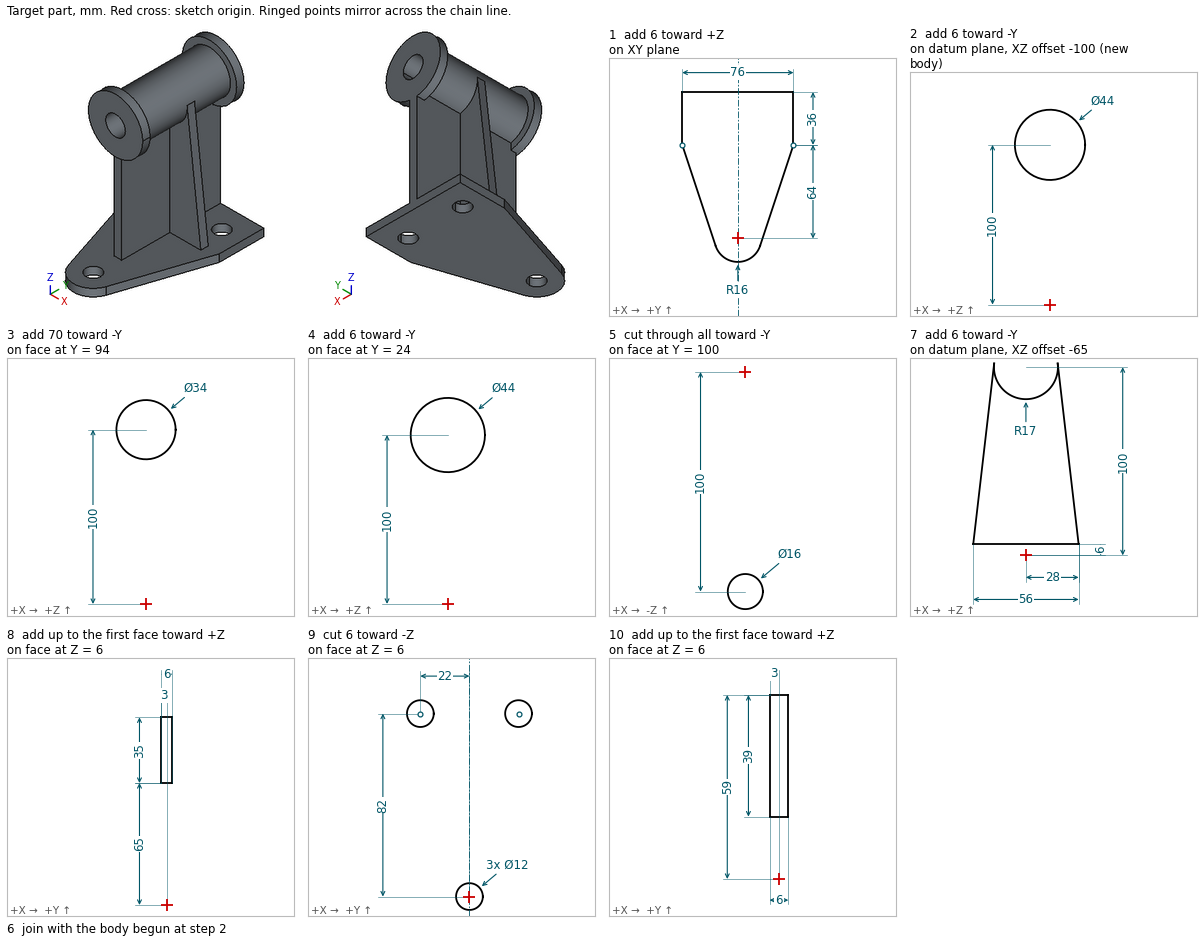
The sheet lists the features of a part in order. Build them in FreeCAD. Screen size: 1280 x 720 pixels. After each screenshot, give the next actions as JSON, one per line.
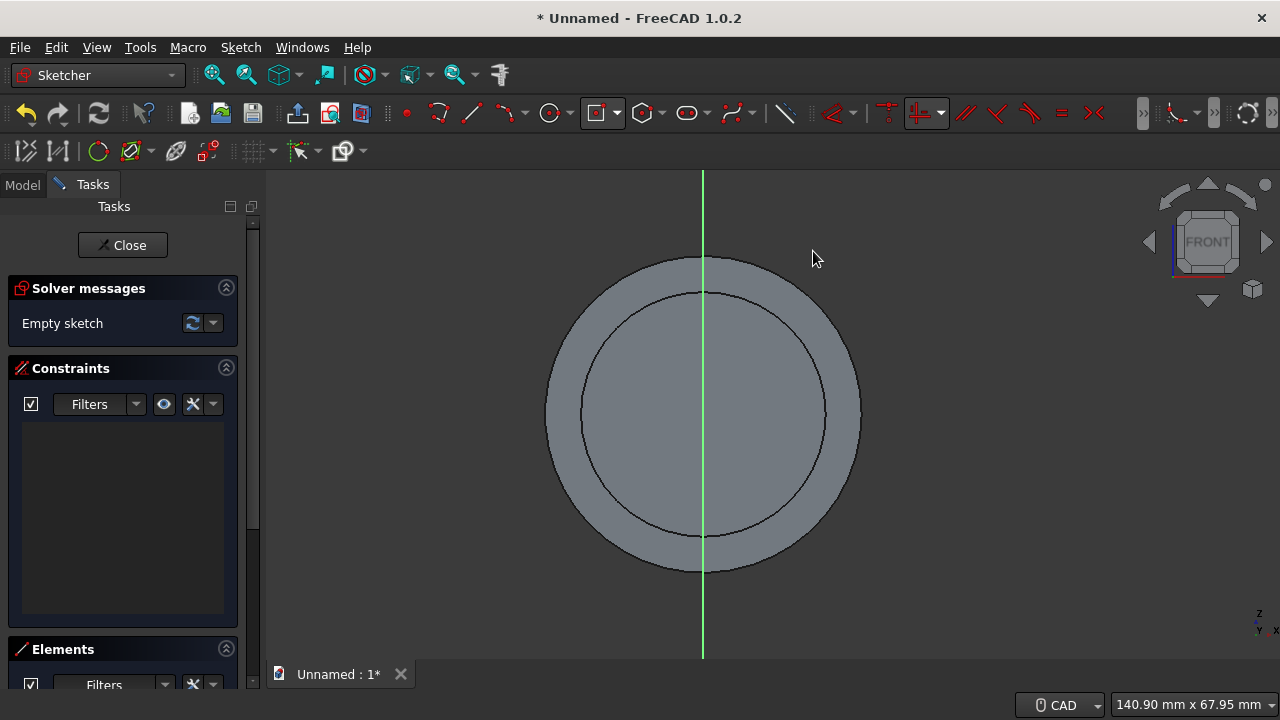
{"action": "key", "text": "g c"}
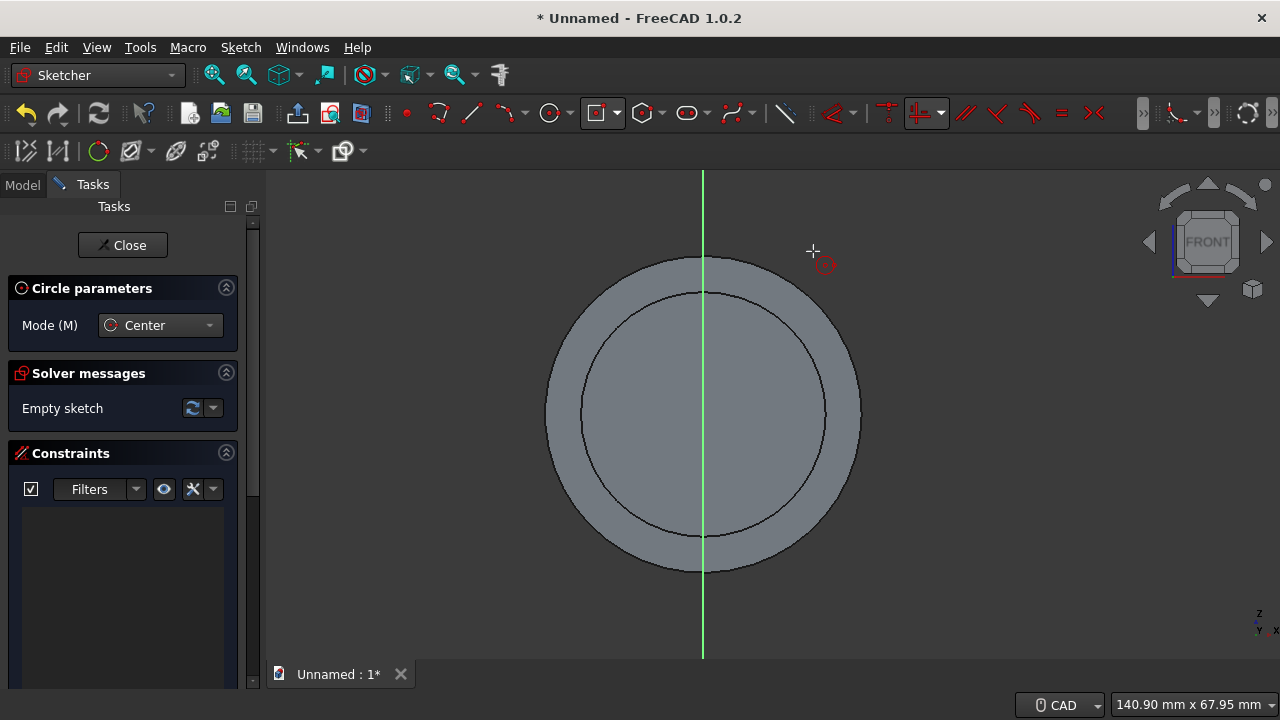
{"action": "left_click", "coordinate": [703, 414]}
{"action": "left_click", "coordinate": [815, 302]}
{"action": "key", "text": "Escape"}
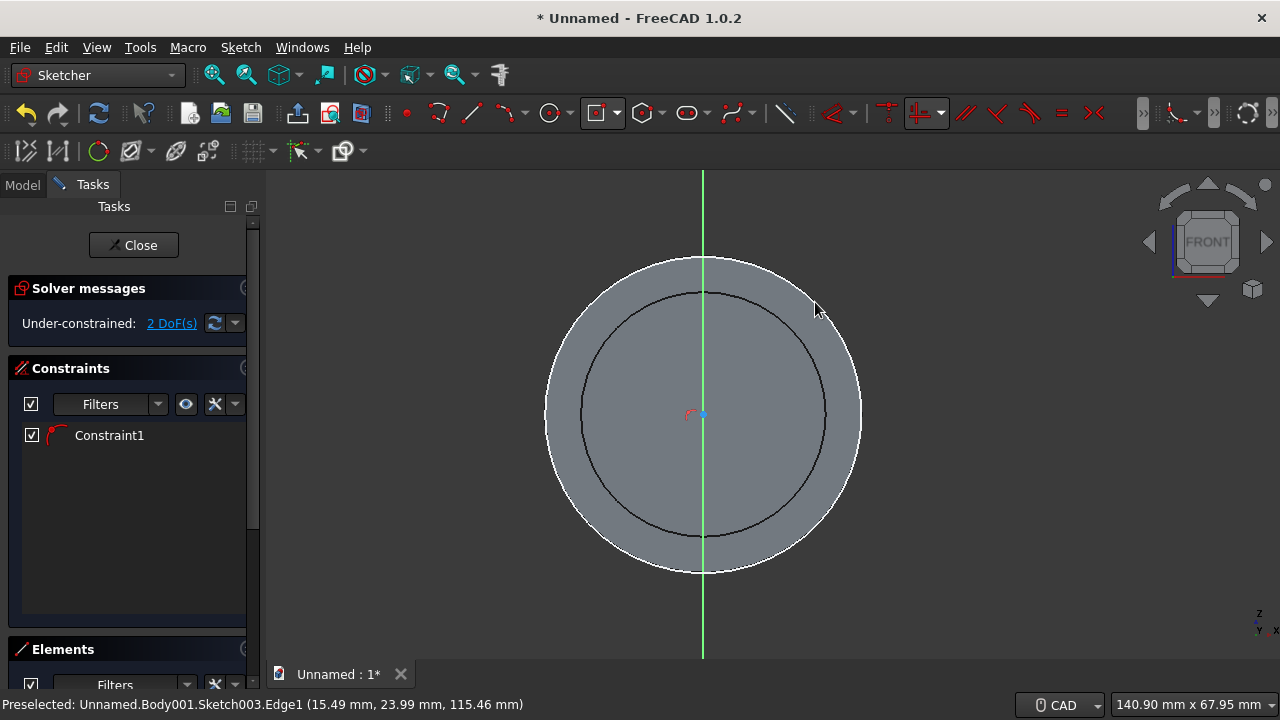
{"action": "key", "text": "d"}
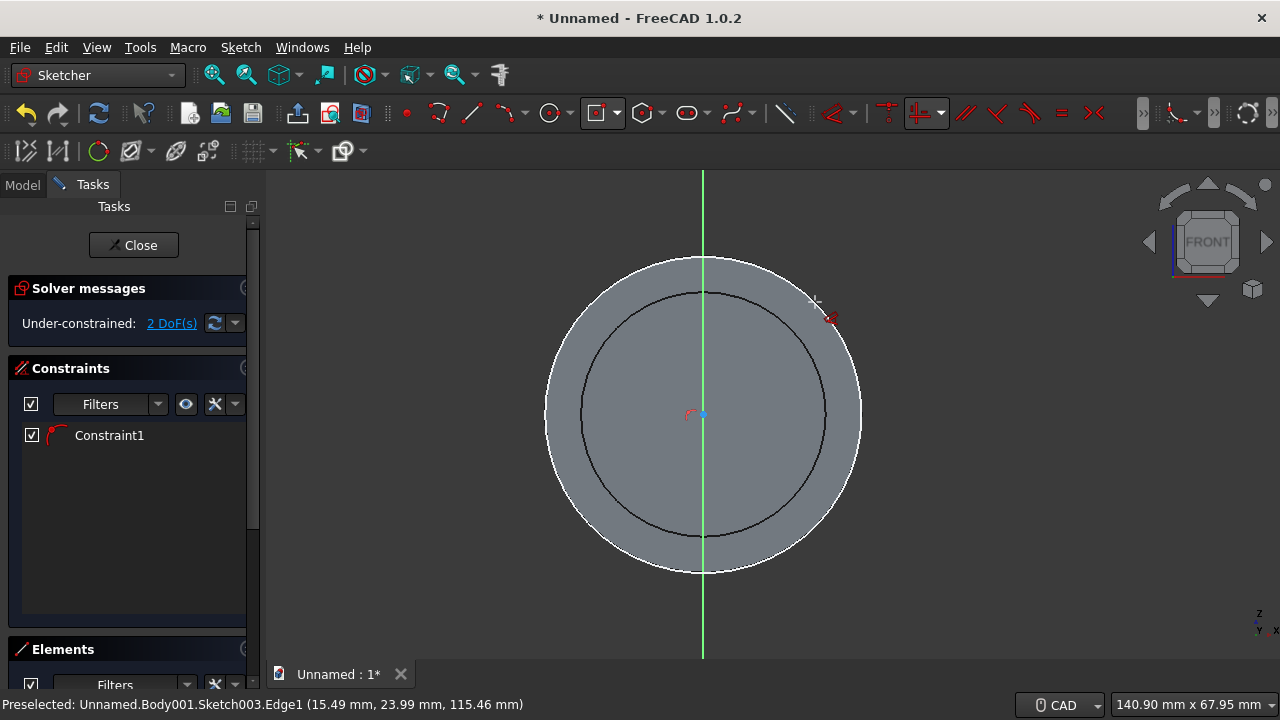
{"action": "left_click", "coordinate": [815, 303]}
{"action": "left_click", "coordinate": [838, 280]}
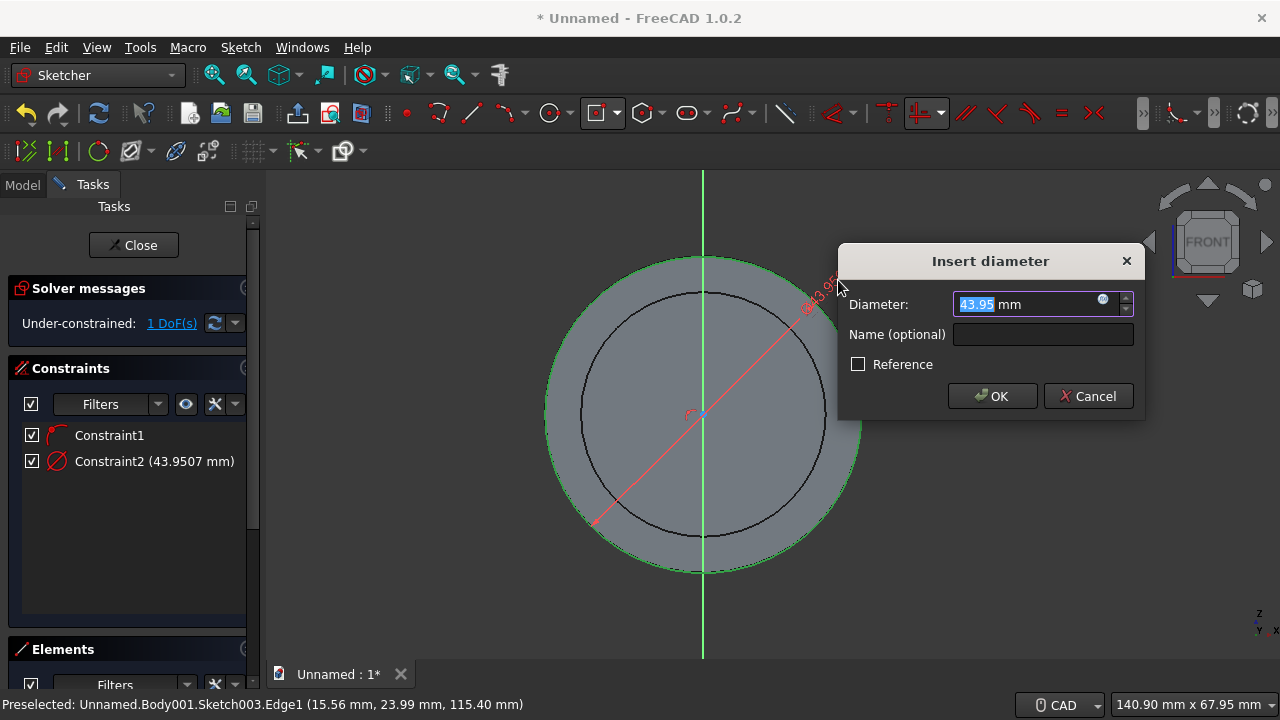
{"action": "type", "text": "44"}
{"action": "key", "text": "Return"}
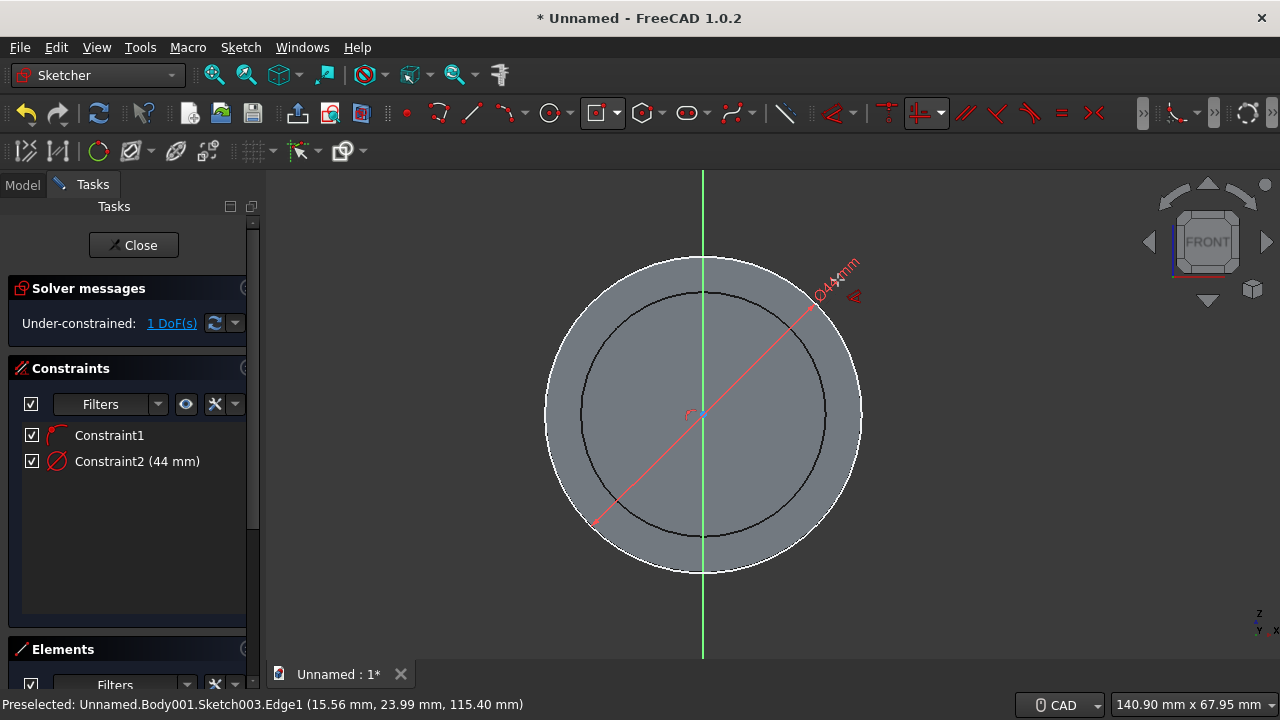
{"action": "left_click", "coordinate": [703, 415]}
{"action": "left_click", "coordinate": [737, 523]}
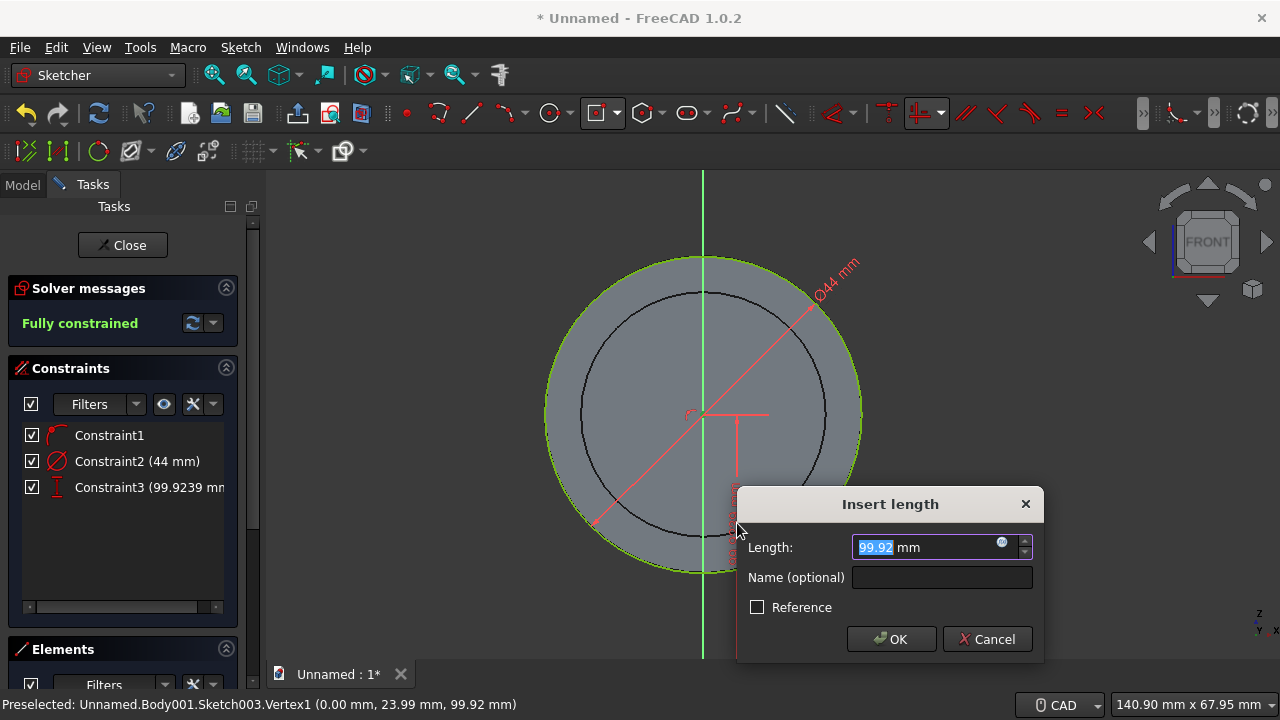
{"action": "type", "text": "100"}
{"action": "key", "text": "Return"}
{"action": "key", "text": "Escape"}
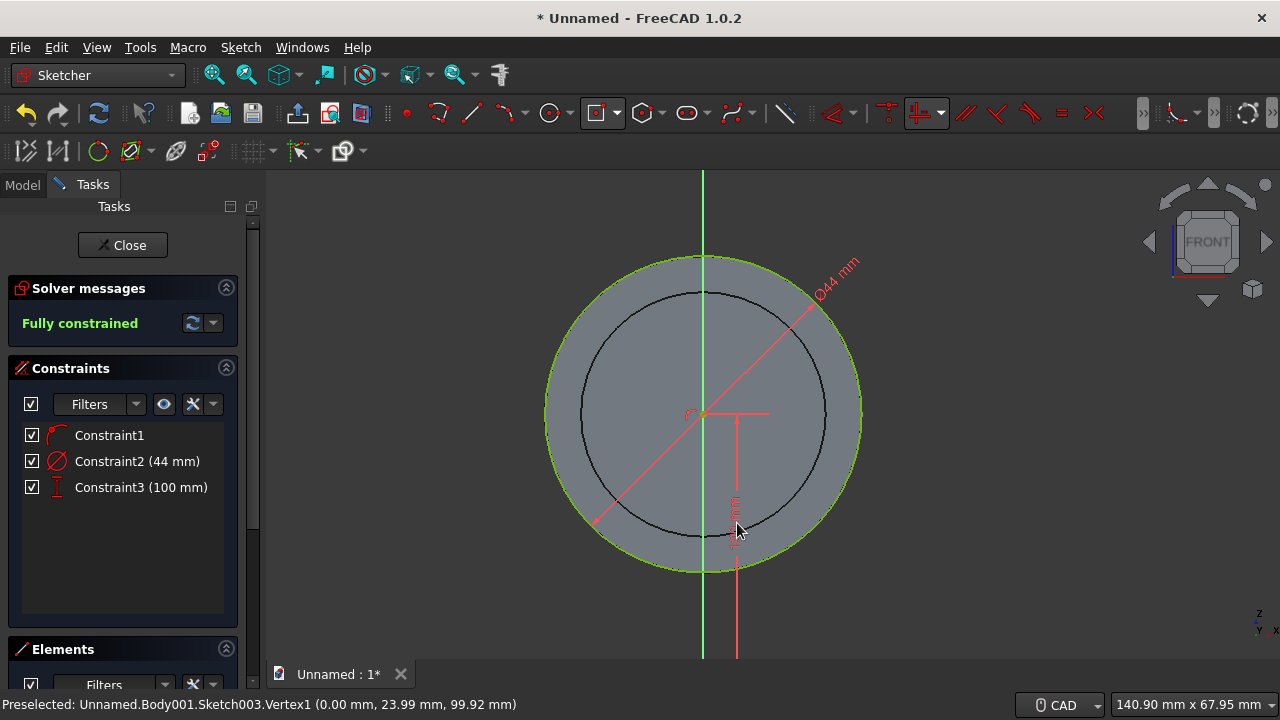
{"action": "left_click", "coordinate": [123, 245]}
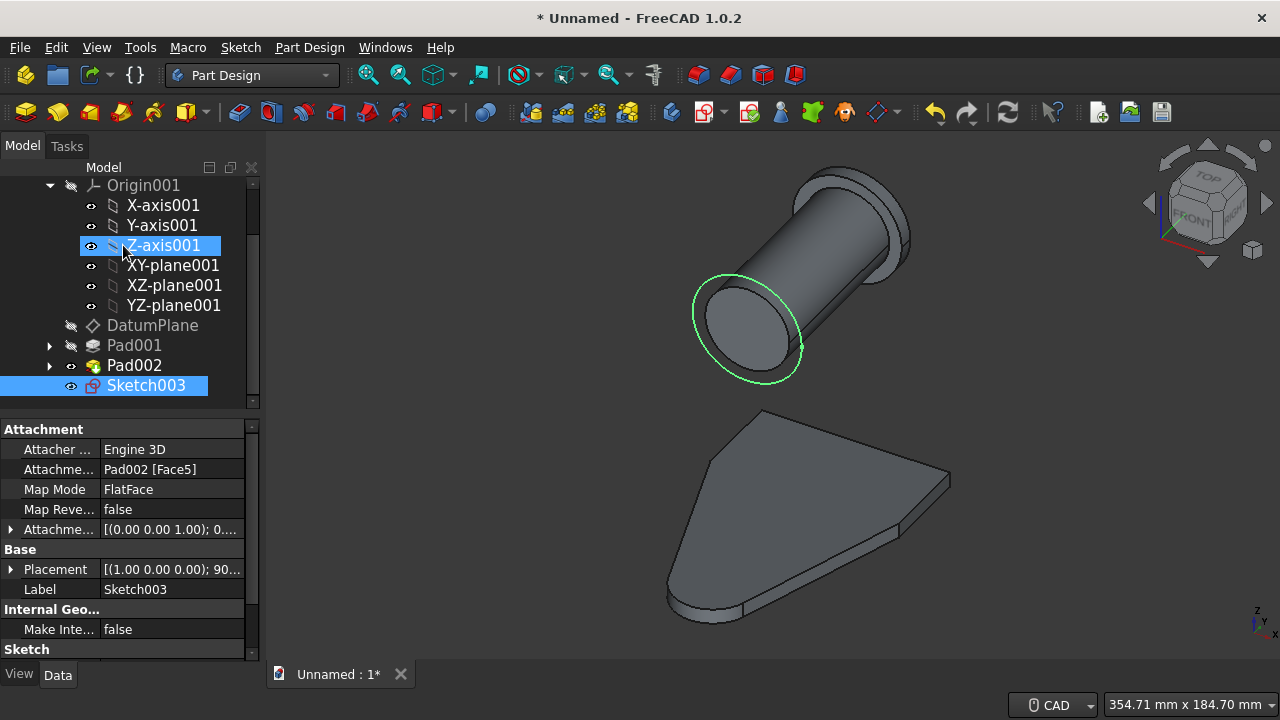
{"action": "left_click", "coordinate": [26, 112]}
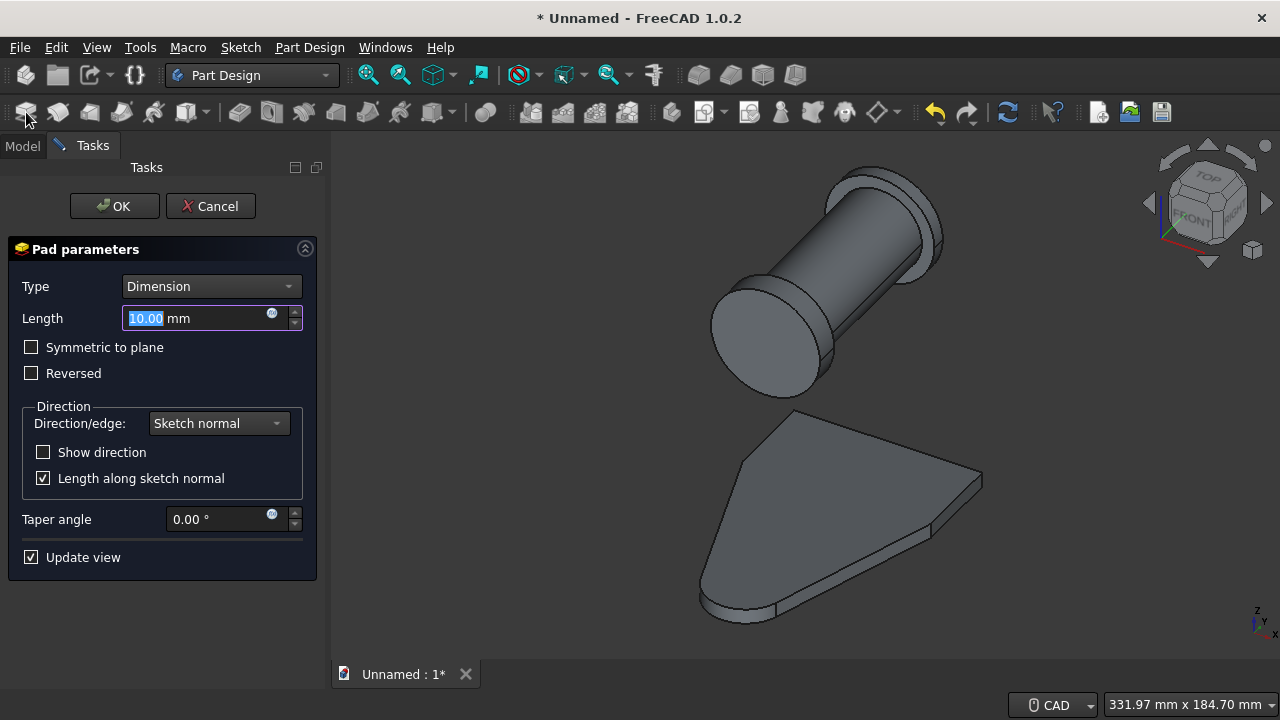
{"action": "type", "text": "6"}
{"action": "key", "text": "Tab"}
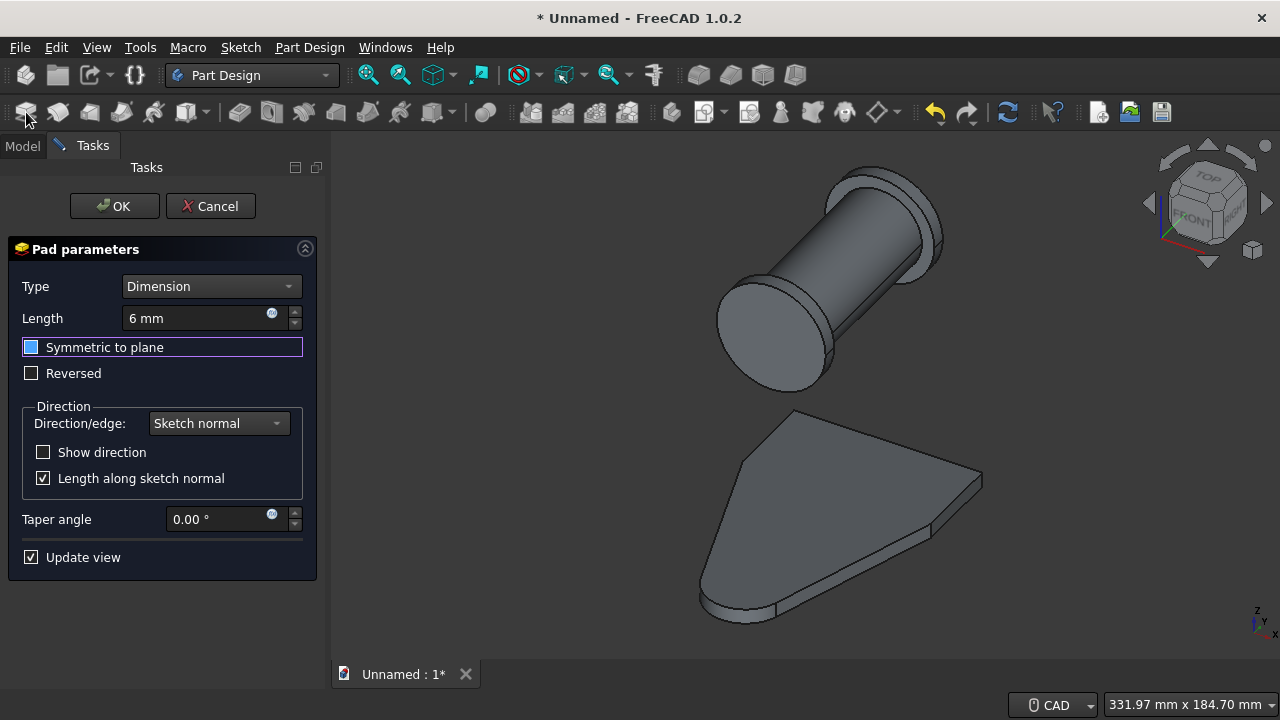
{"action": "left_click", "coordinate": [115, 206]}